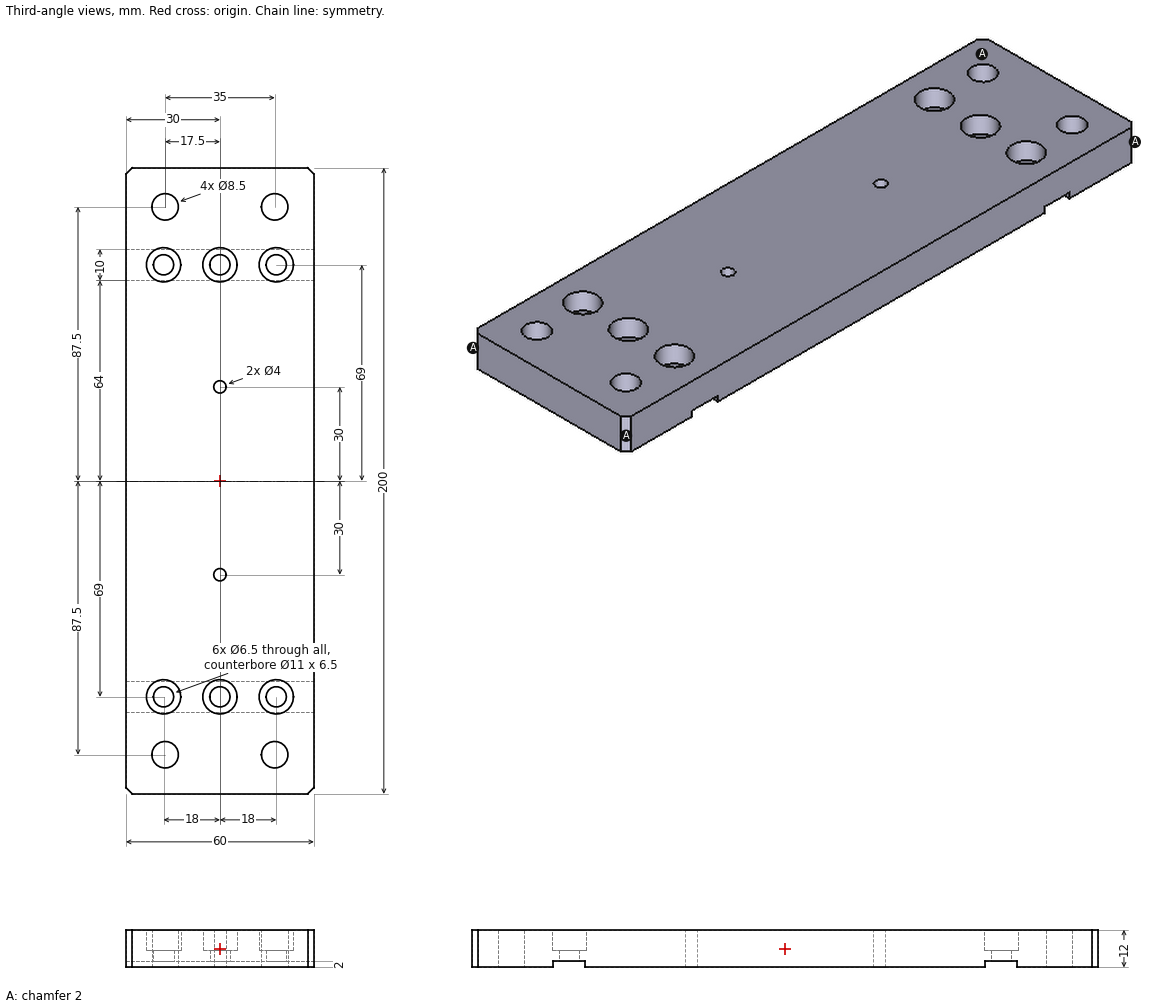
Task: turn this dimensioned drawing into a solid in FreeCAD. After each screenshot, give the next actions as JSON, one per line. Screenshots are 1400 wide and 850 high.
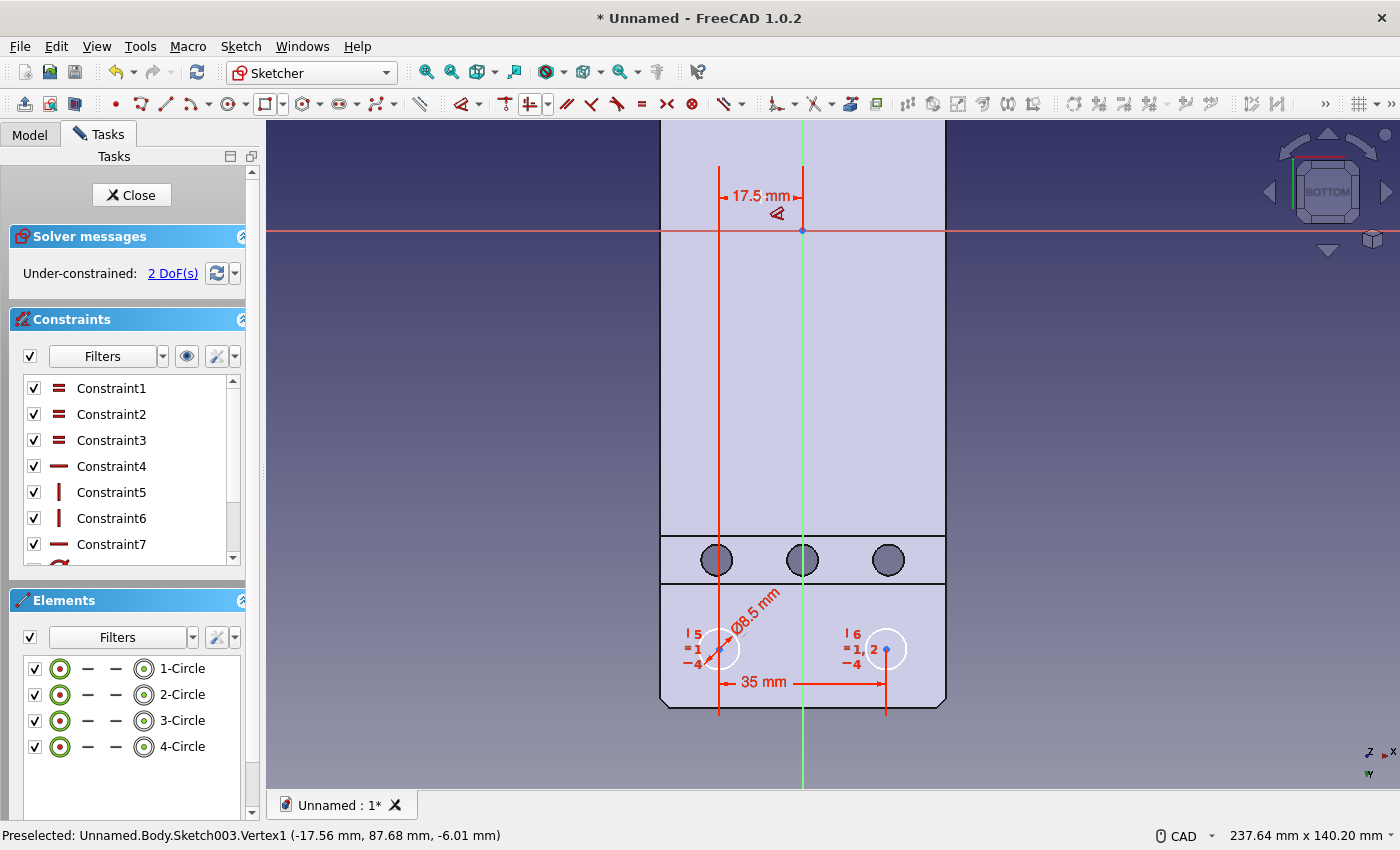
{"action": "left_click", "coordinate": [719, 649]}
{"action": "left_click", "coordinate": [685, 440]}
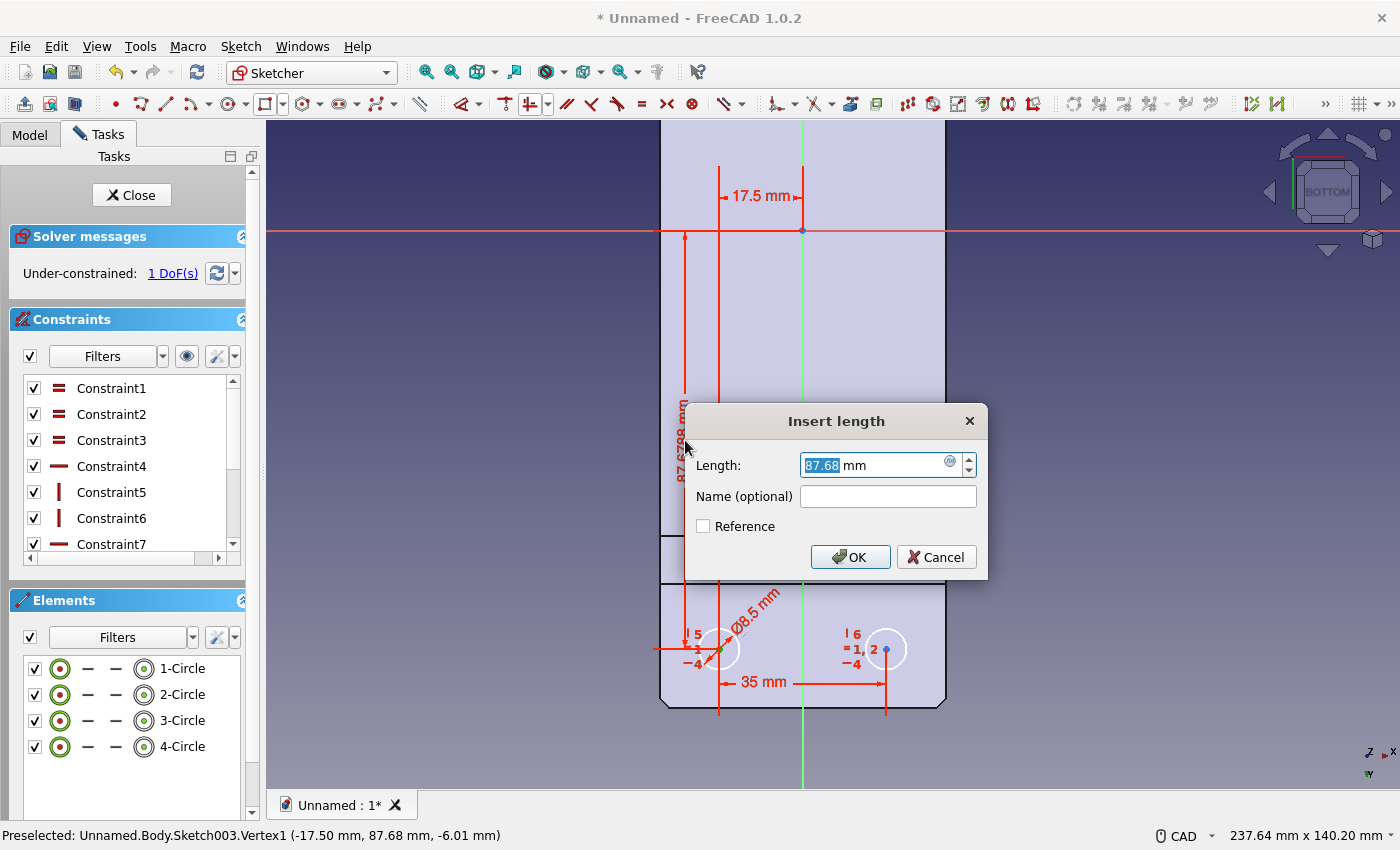
{"action": "type", "text": "87.5"}
{"action": "key", "text": "Return"}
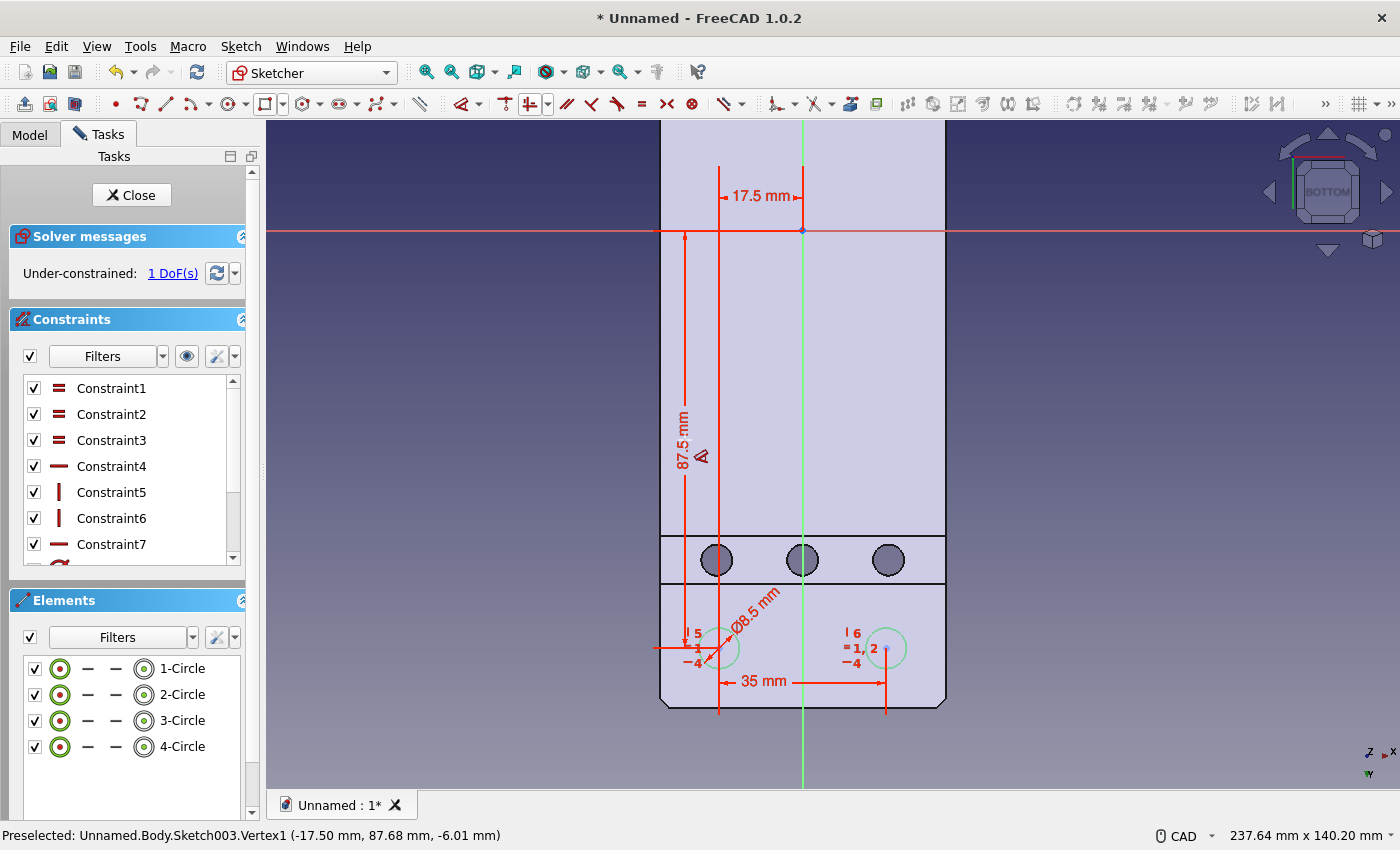
{"action": "scroll", "coordinate": [733, 637], "scroll_direction": "down", "scroll_amount": 4}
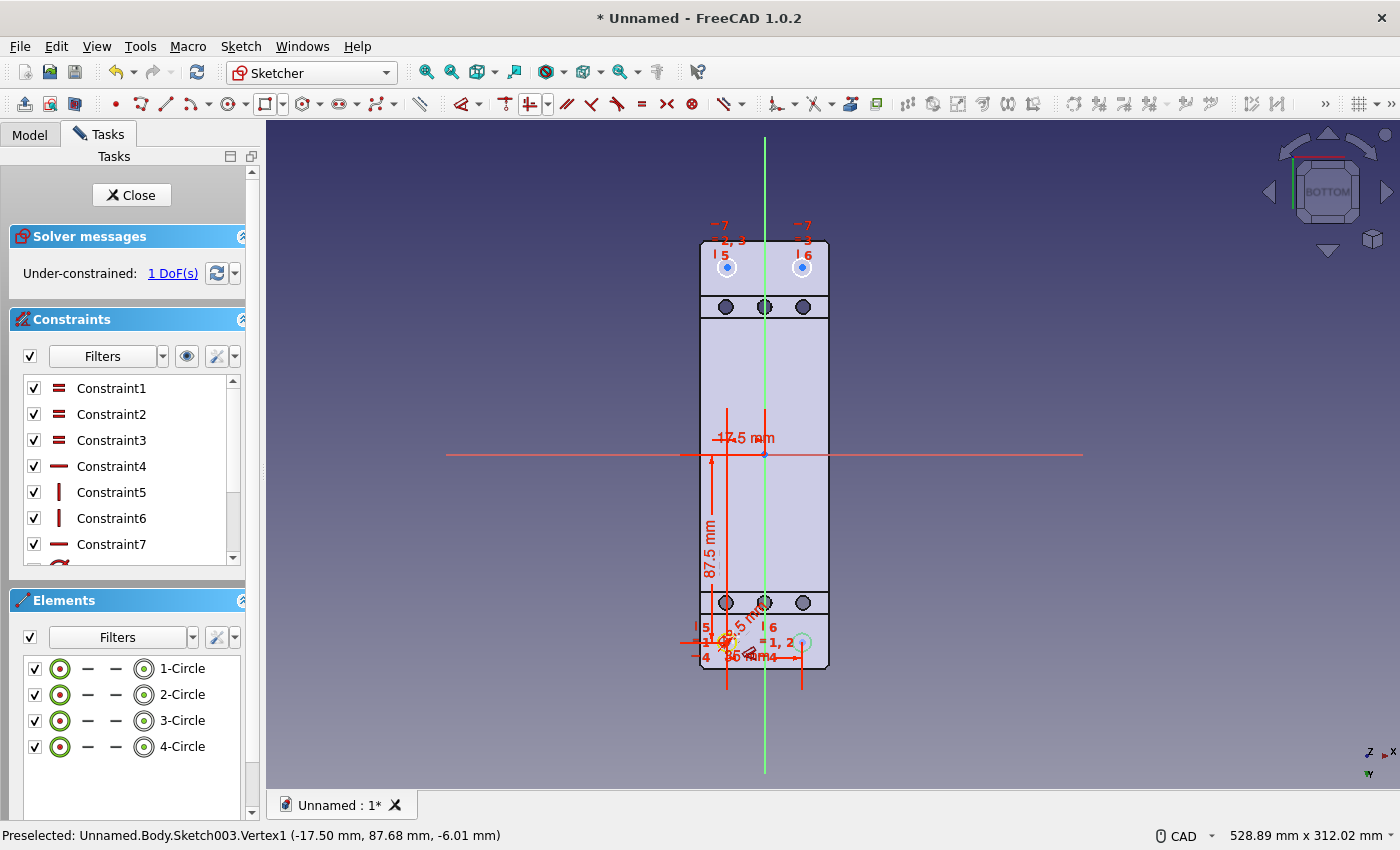
{"action": "left_click", "coordinate": [727, 268]}
{"action": "left_click", "coordinate": [693, 361]}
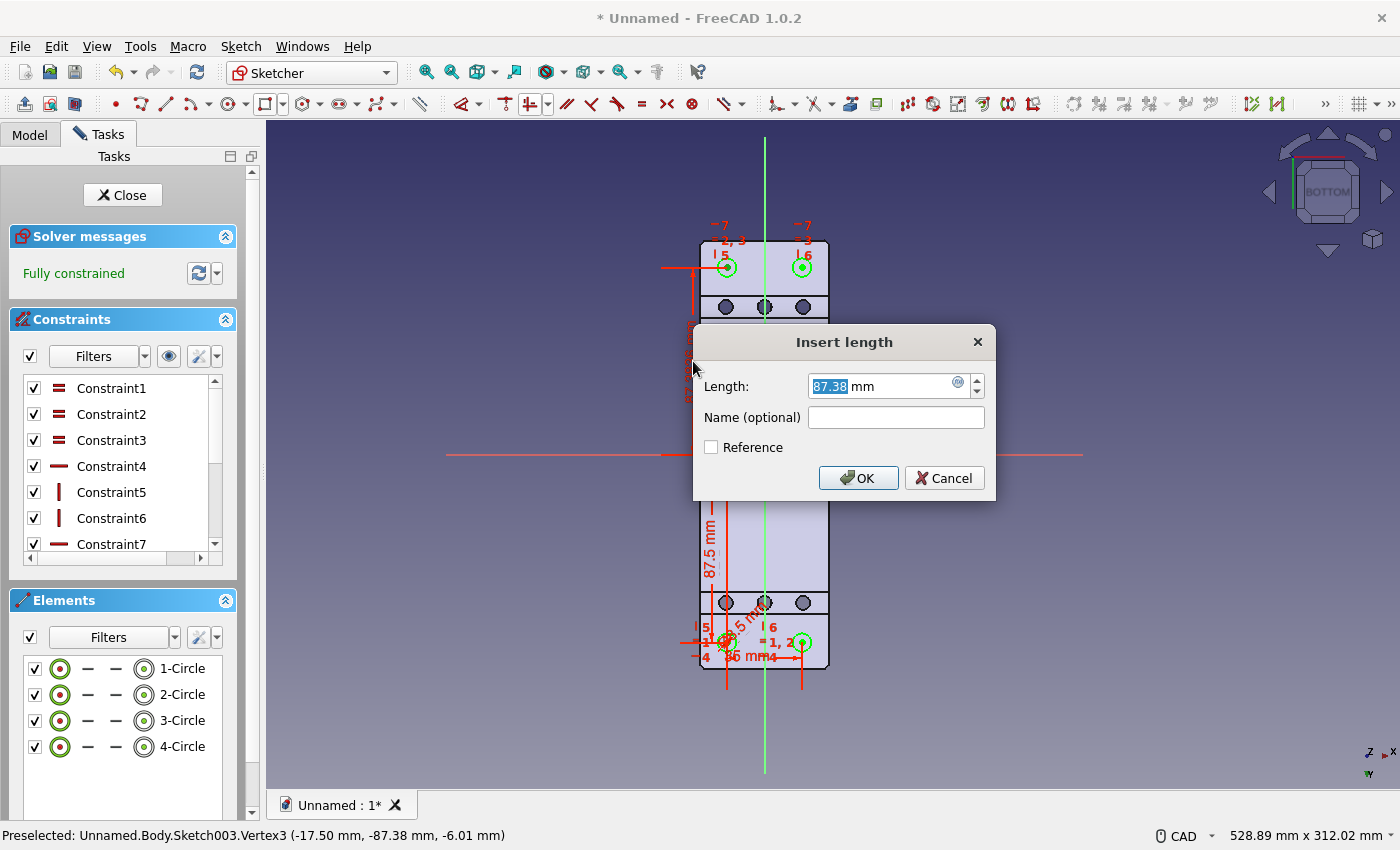
{"action": "type", "text": "87.5"}
{"action": "key", "text": "Return"}
{"action": "key", "text": "Escape"}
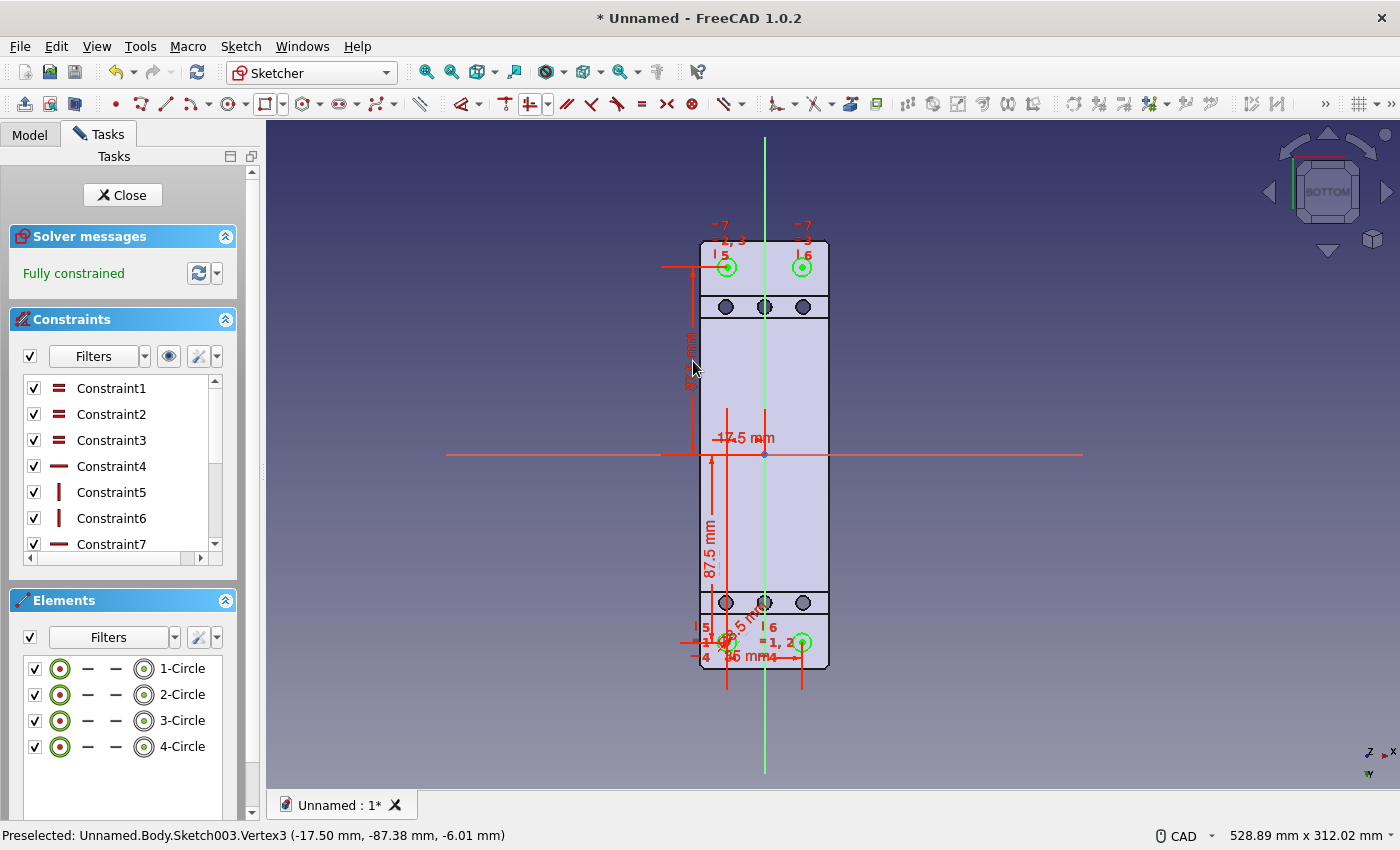
{"action": "left_click", "coordinate": [123, 195]}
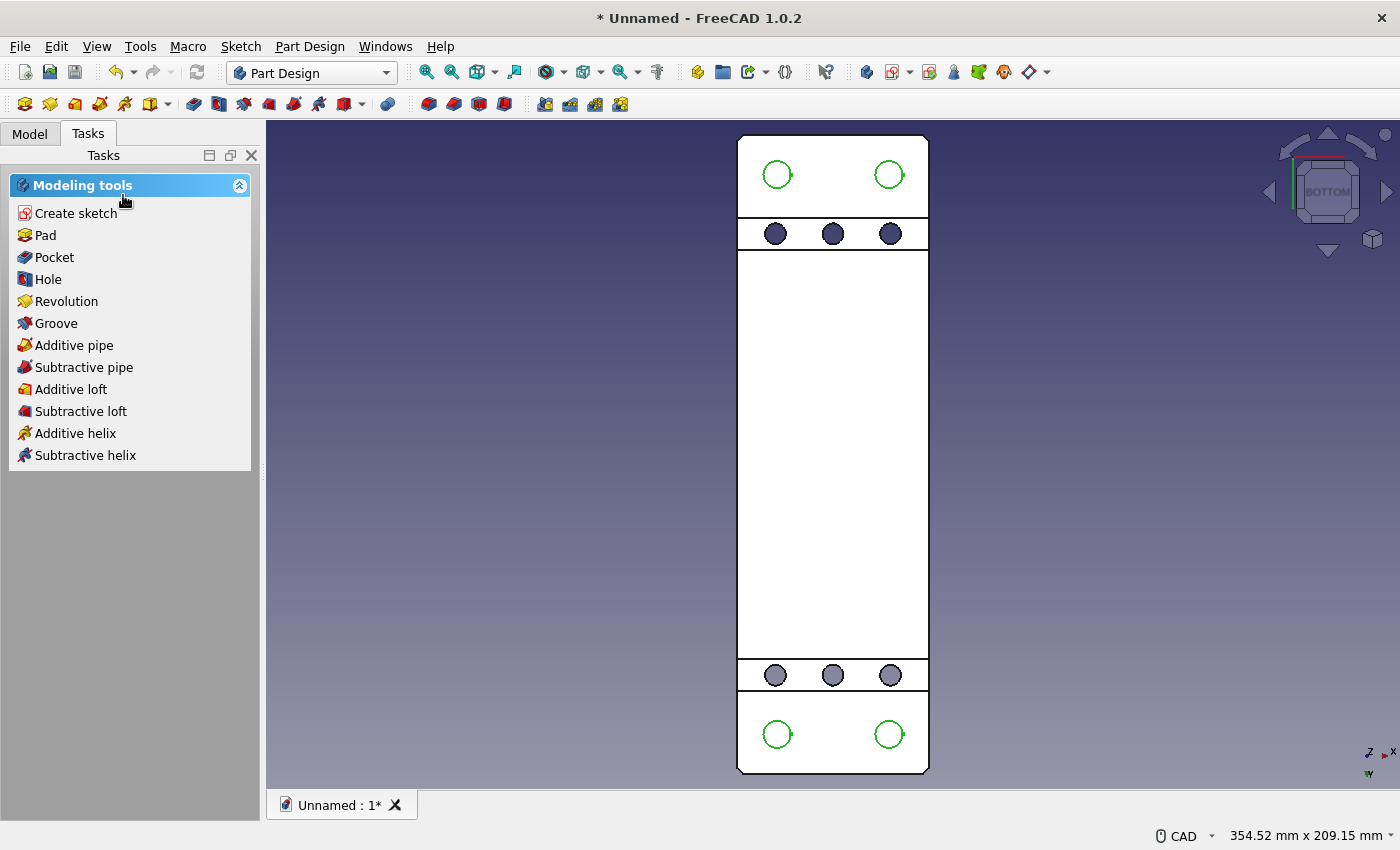
{"action": "left_click", "coordinate": [194, 104]}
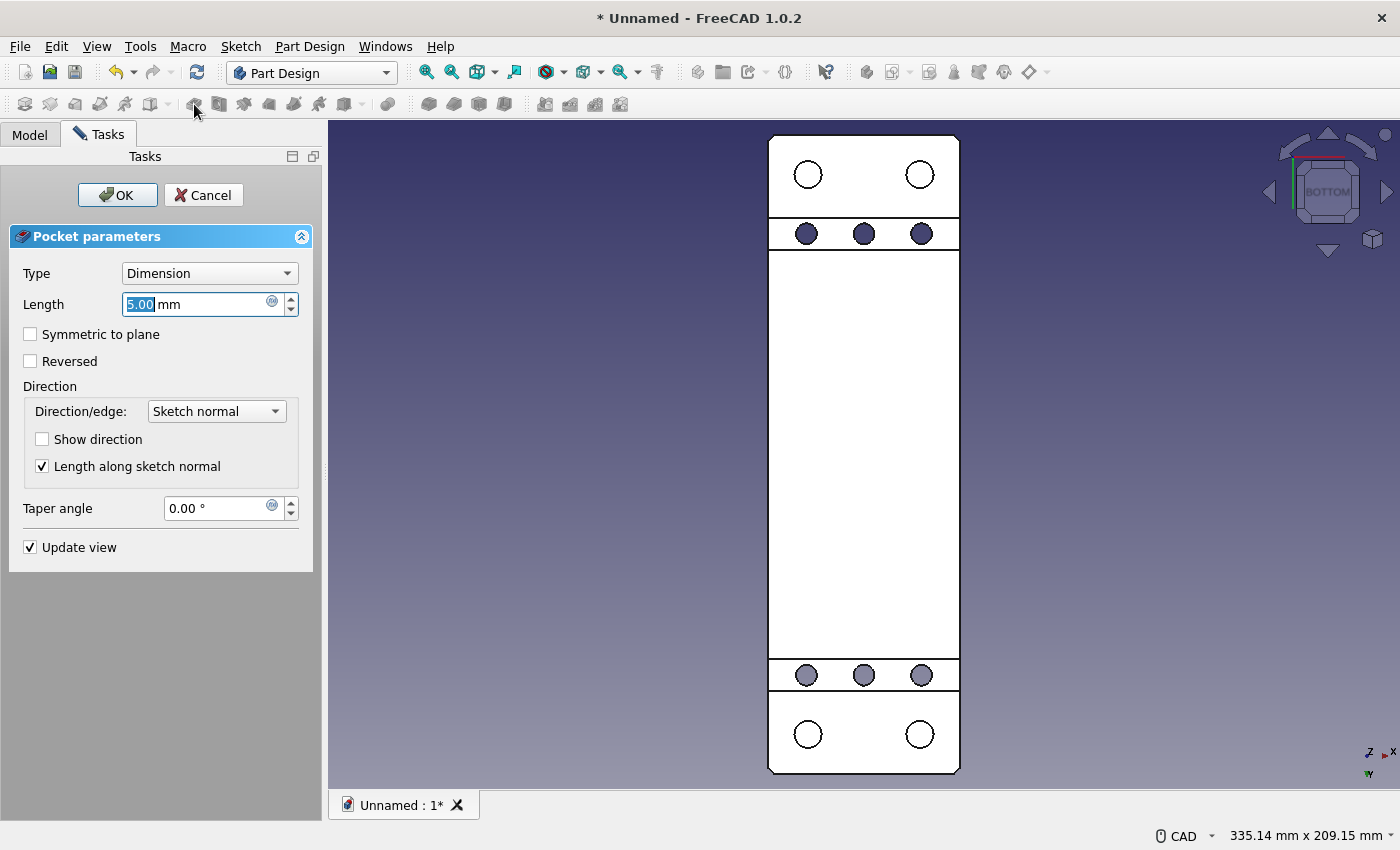
{"action": "left_click", "coordinate": [210, 274]}